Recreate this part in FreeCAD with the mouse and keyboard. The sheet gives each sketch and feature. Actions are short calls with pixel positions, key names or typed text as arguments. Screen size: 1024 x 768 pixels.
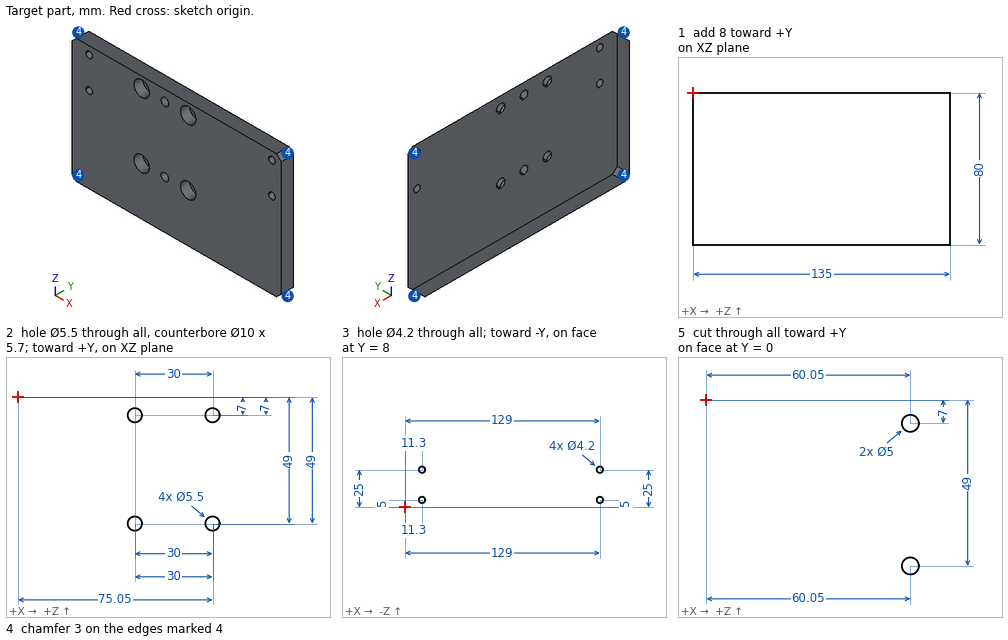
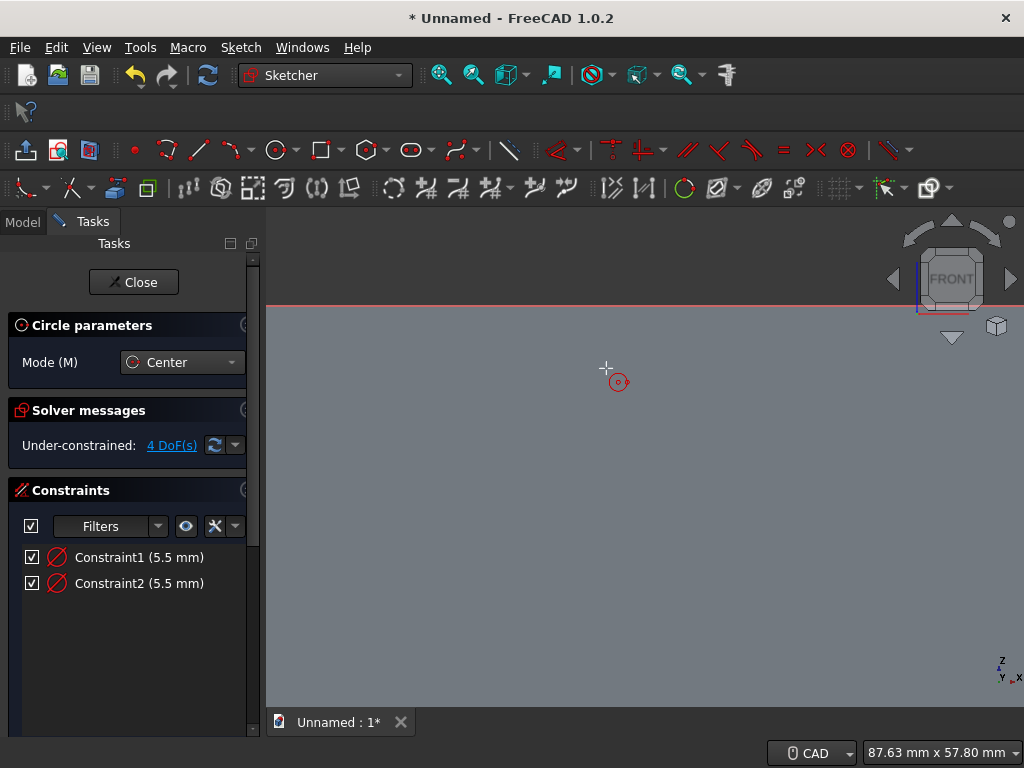
click(606, 367)
move(623, 350)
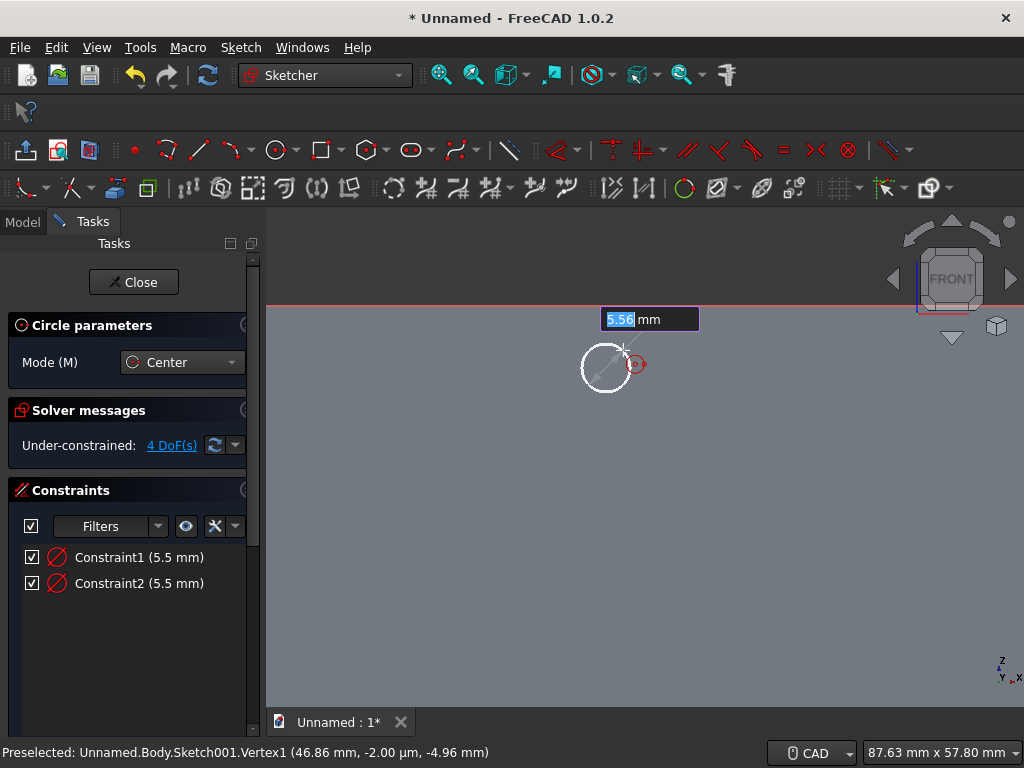
text(5.5)
key(Return)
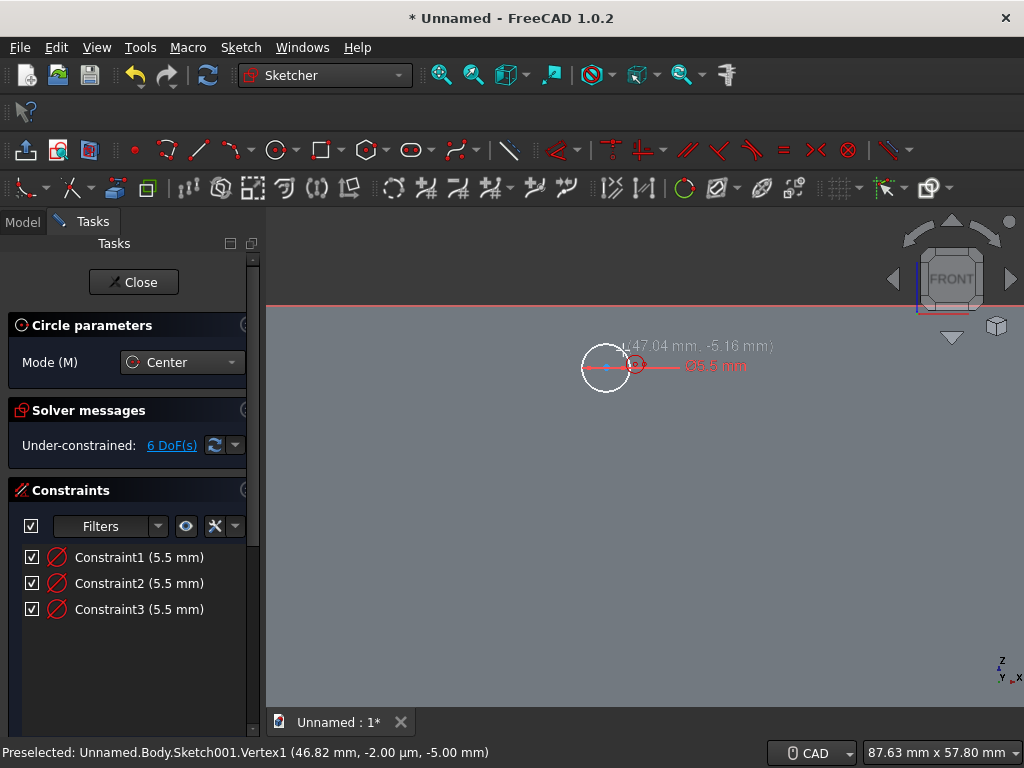
scroll(606, 368, down, 3)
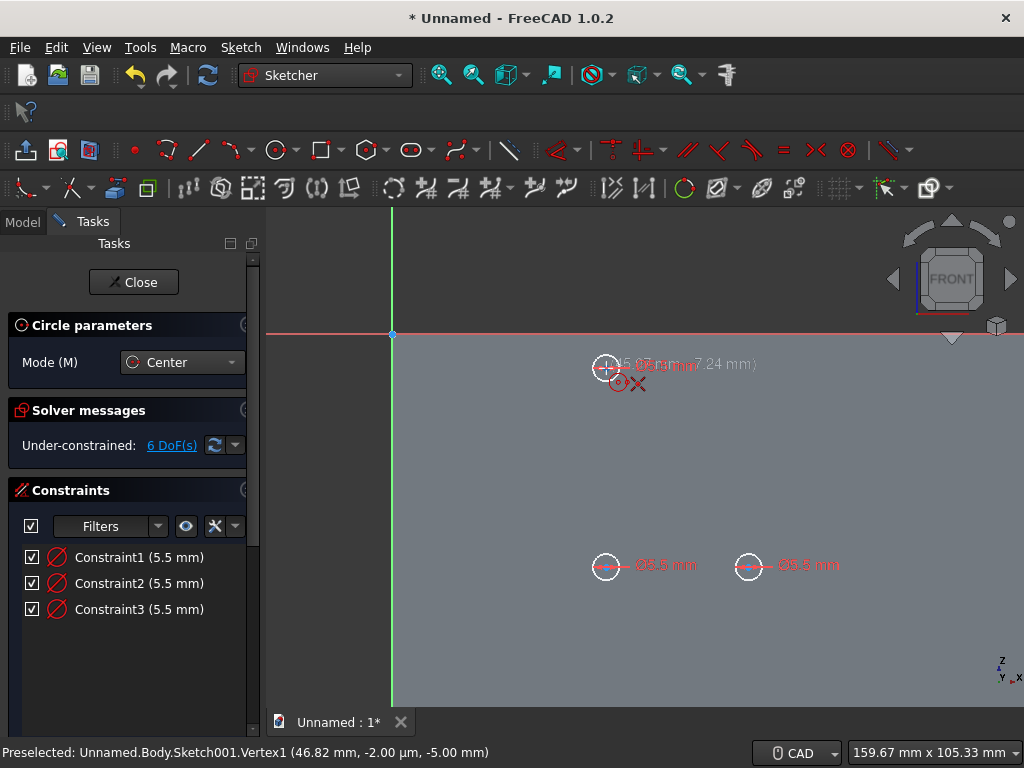
scroll(749, 368, up, 3)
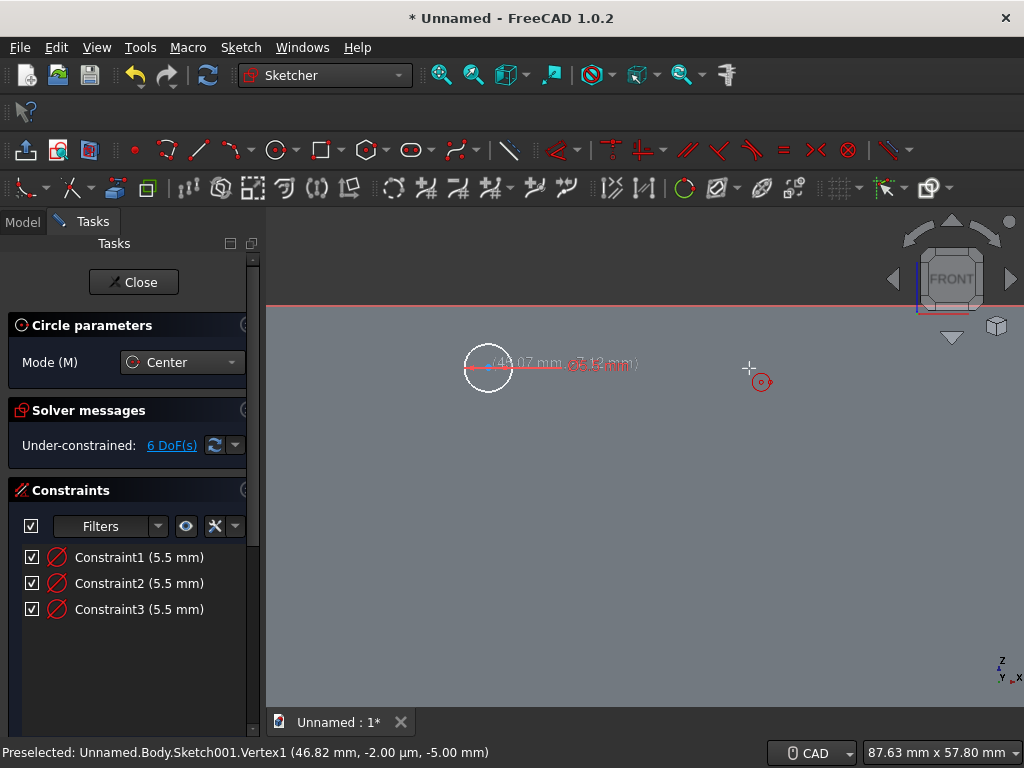
click(748, 367)
move(764, 350)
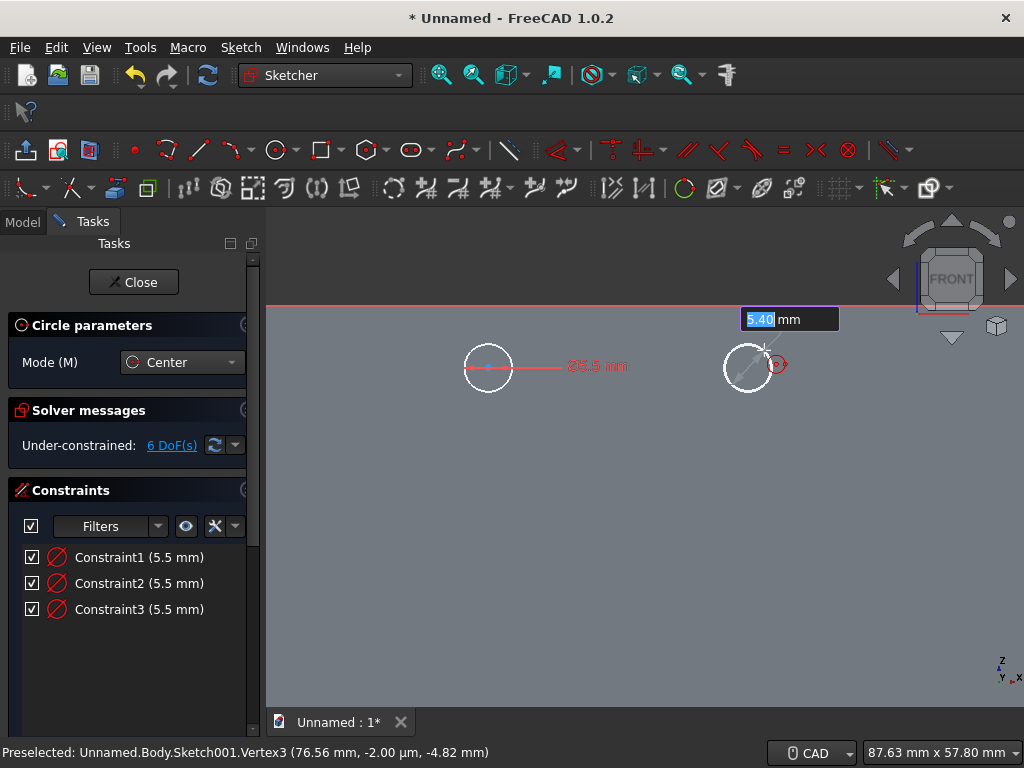
text(5.5)
key(Return)
key(Escape)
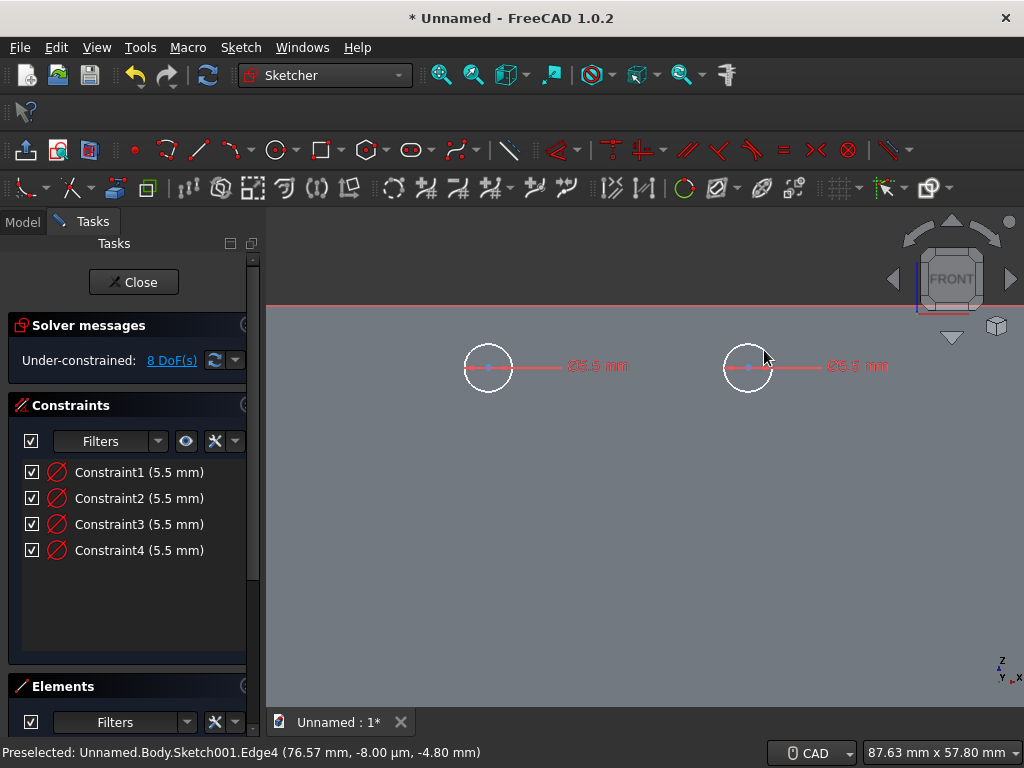
click(488, 368)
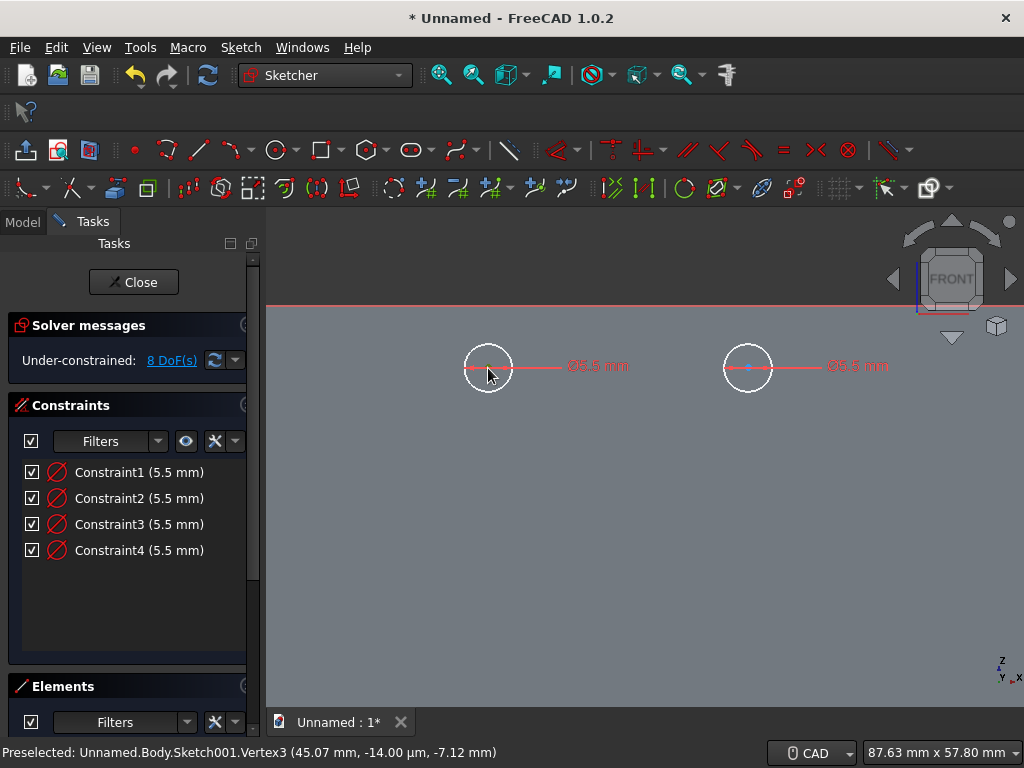
key(i)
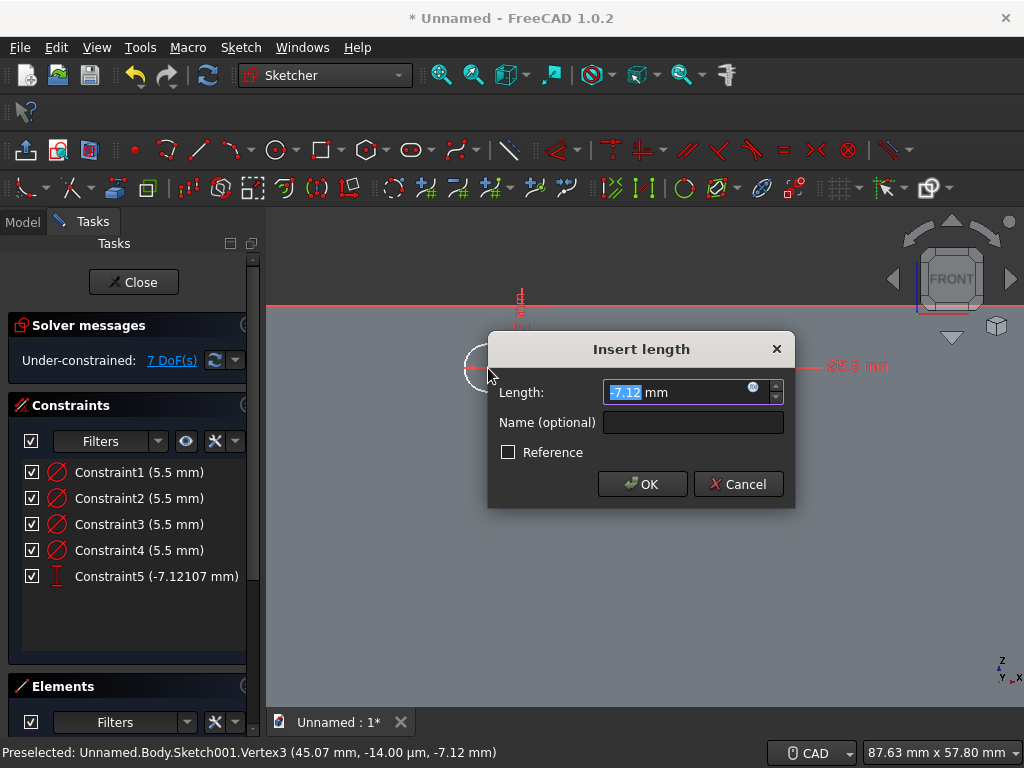
text(-7)
key(Return)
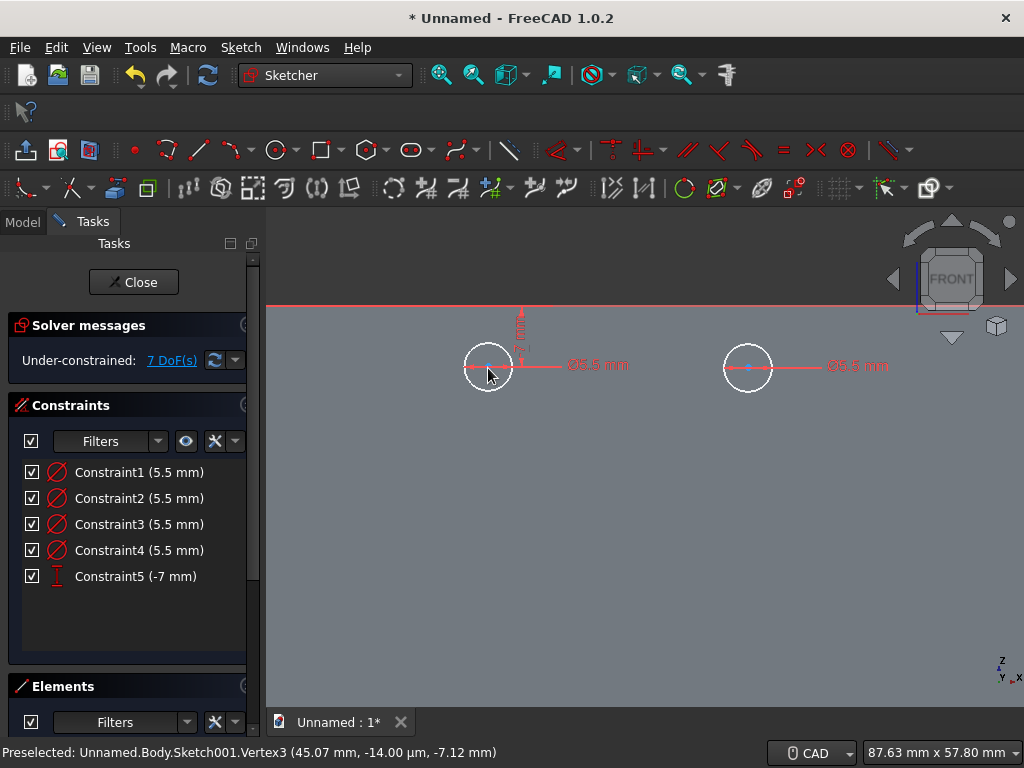
click(748, 368)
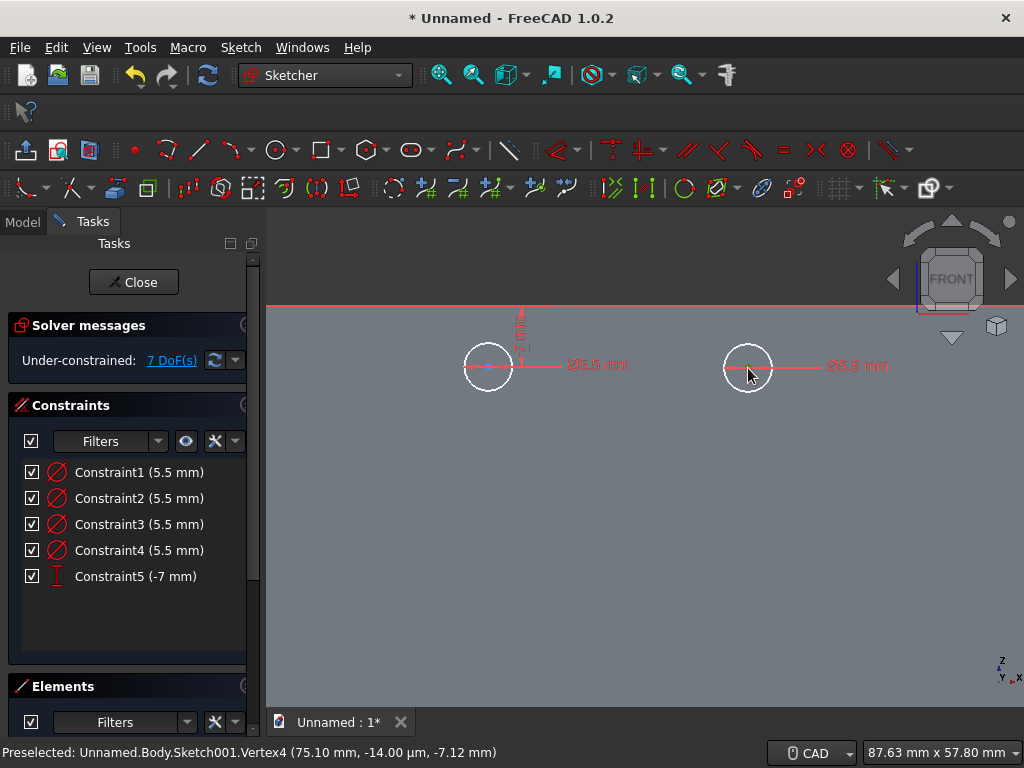
key(i)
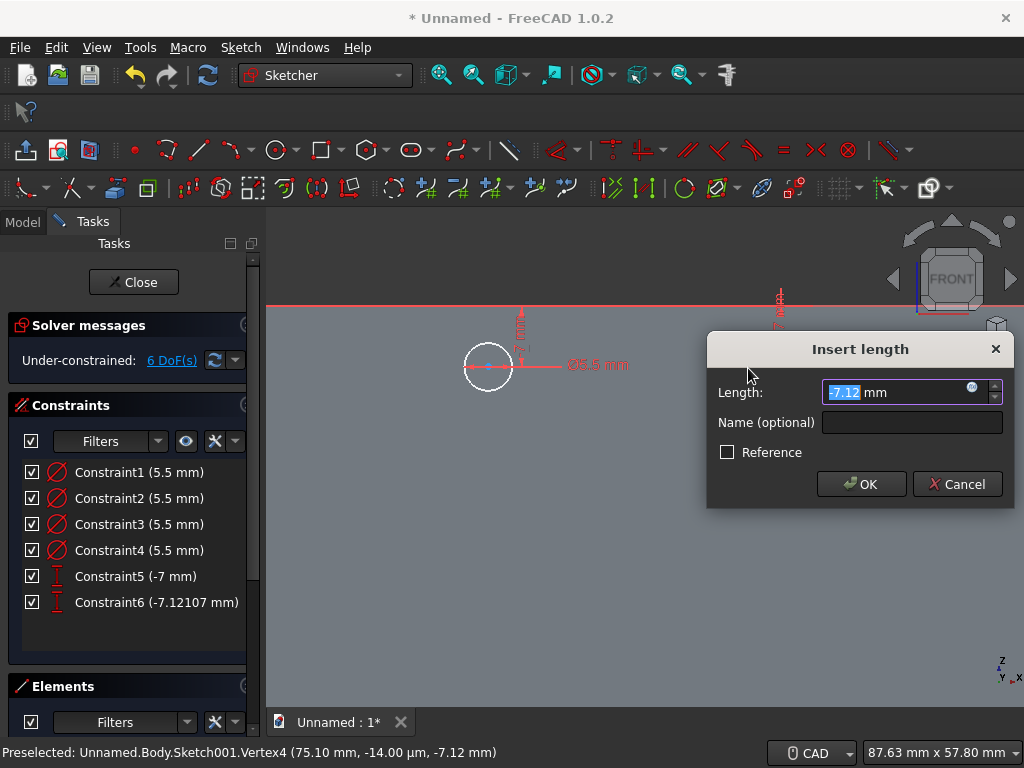
text(-7)
key(Return)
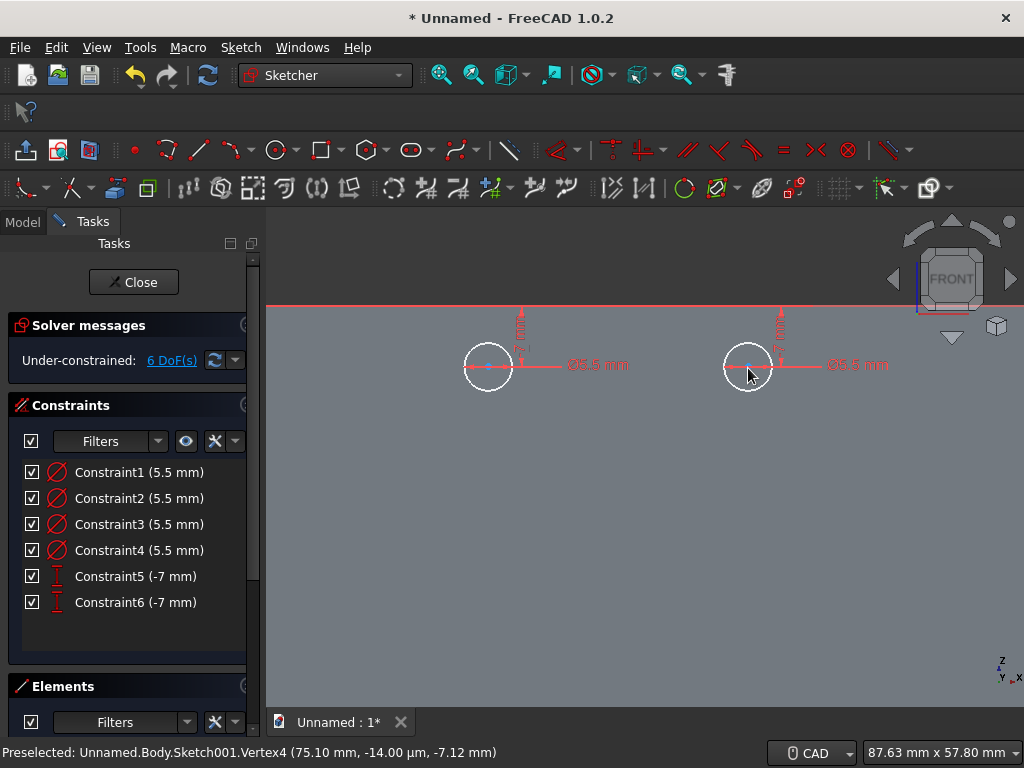
scroll(749, 368, down, 3)